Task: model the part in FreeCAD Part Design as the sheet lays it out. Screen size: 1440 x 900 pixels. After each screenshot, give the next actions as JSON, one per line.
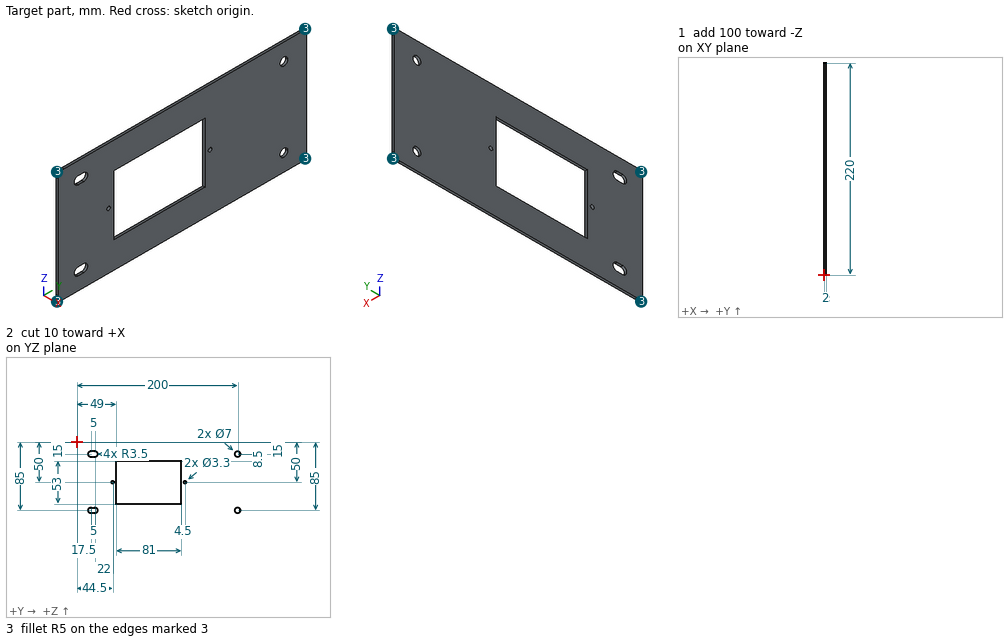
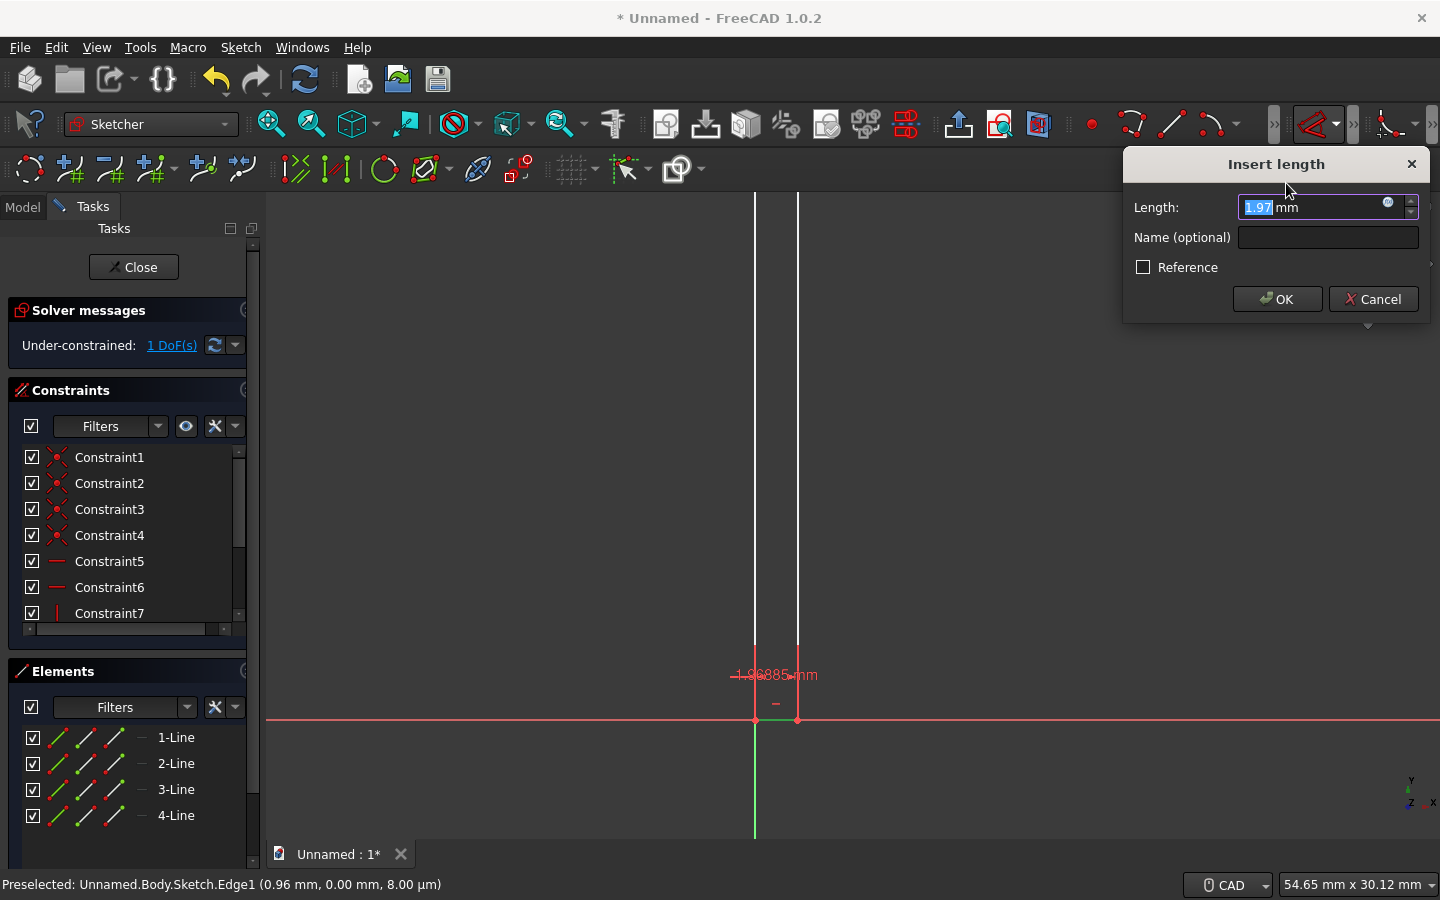
{"action": "type", "text": "2"}
{"action": "key", "text": "Return"}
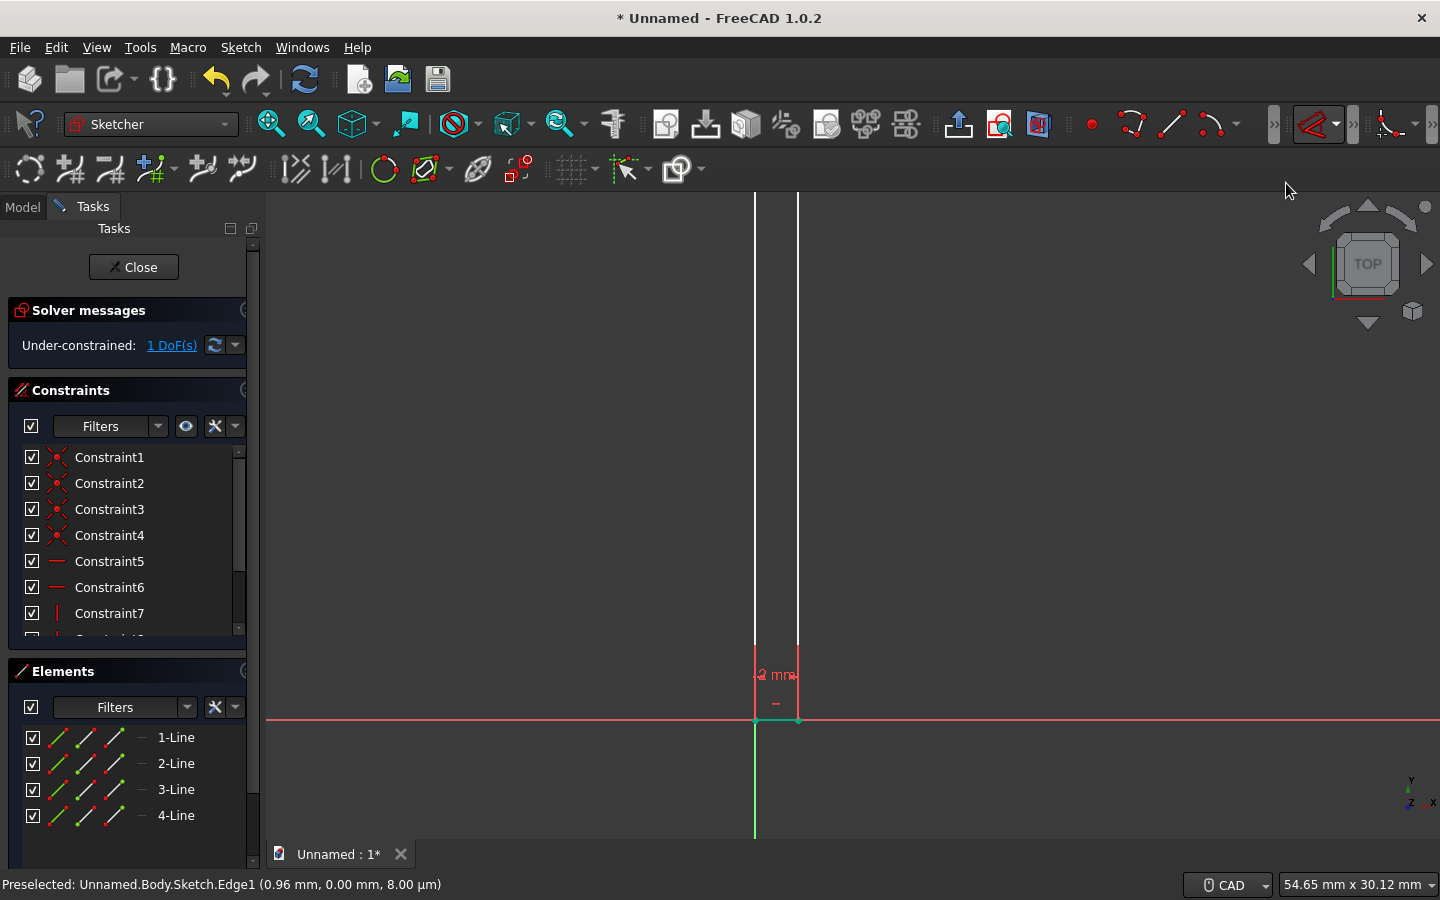
{"action": "scroll", "coordinate": [785, 731], "scroll_direction": "down", "scroll_amount": 12}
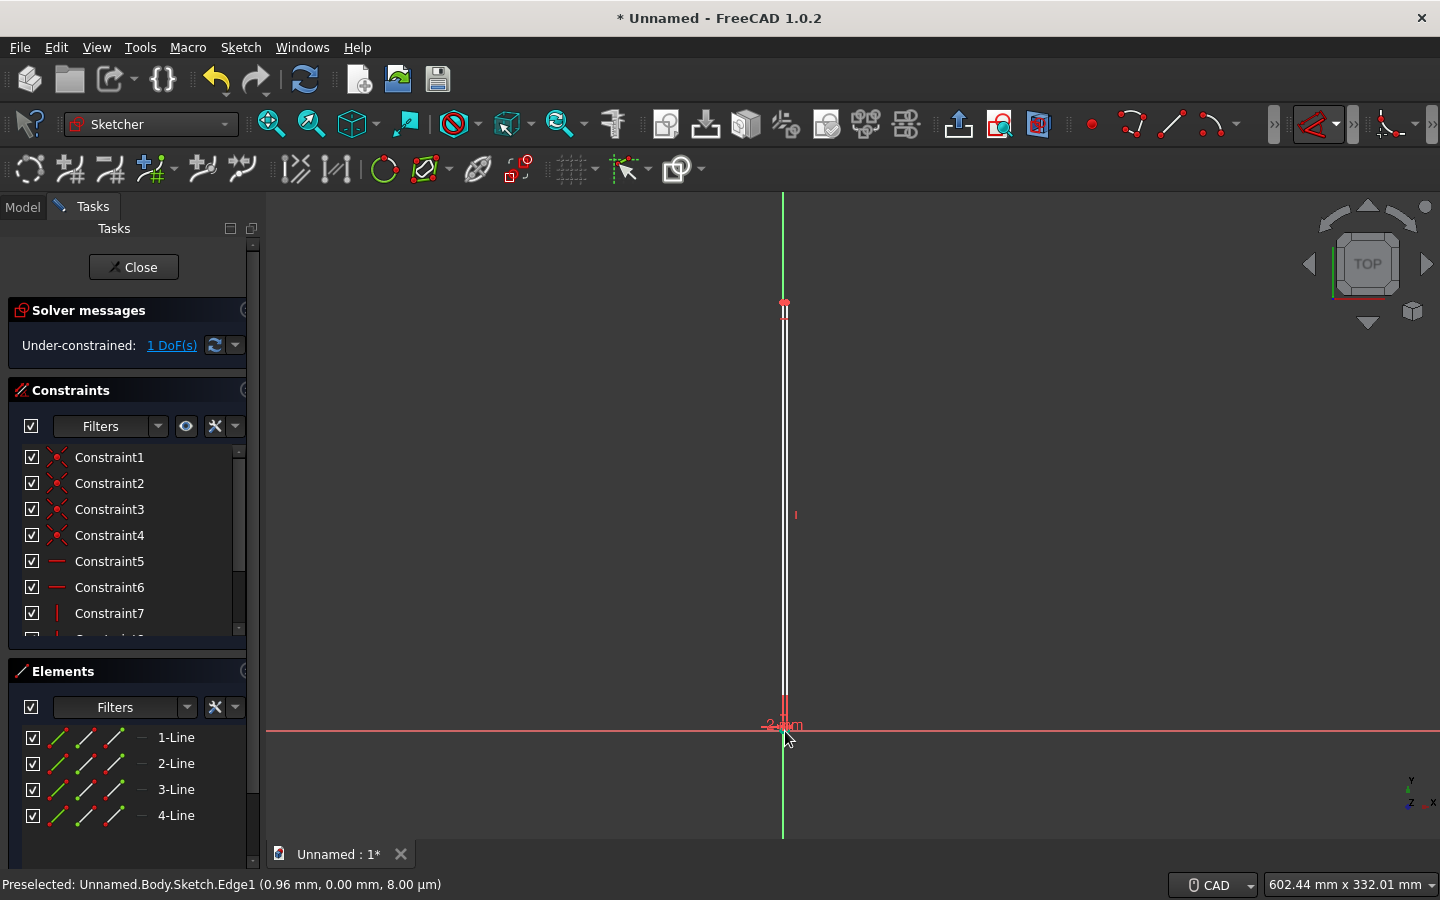
{"action": "scroll", "coordinate": [787, 602], "scroll_direction": "up", "scroll_amount": 7}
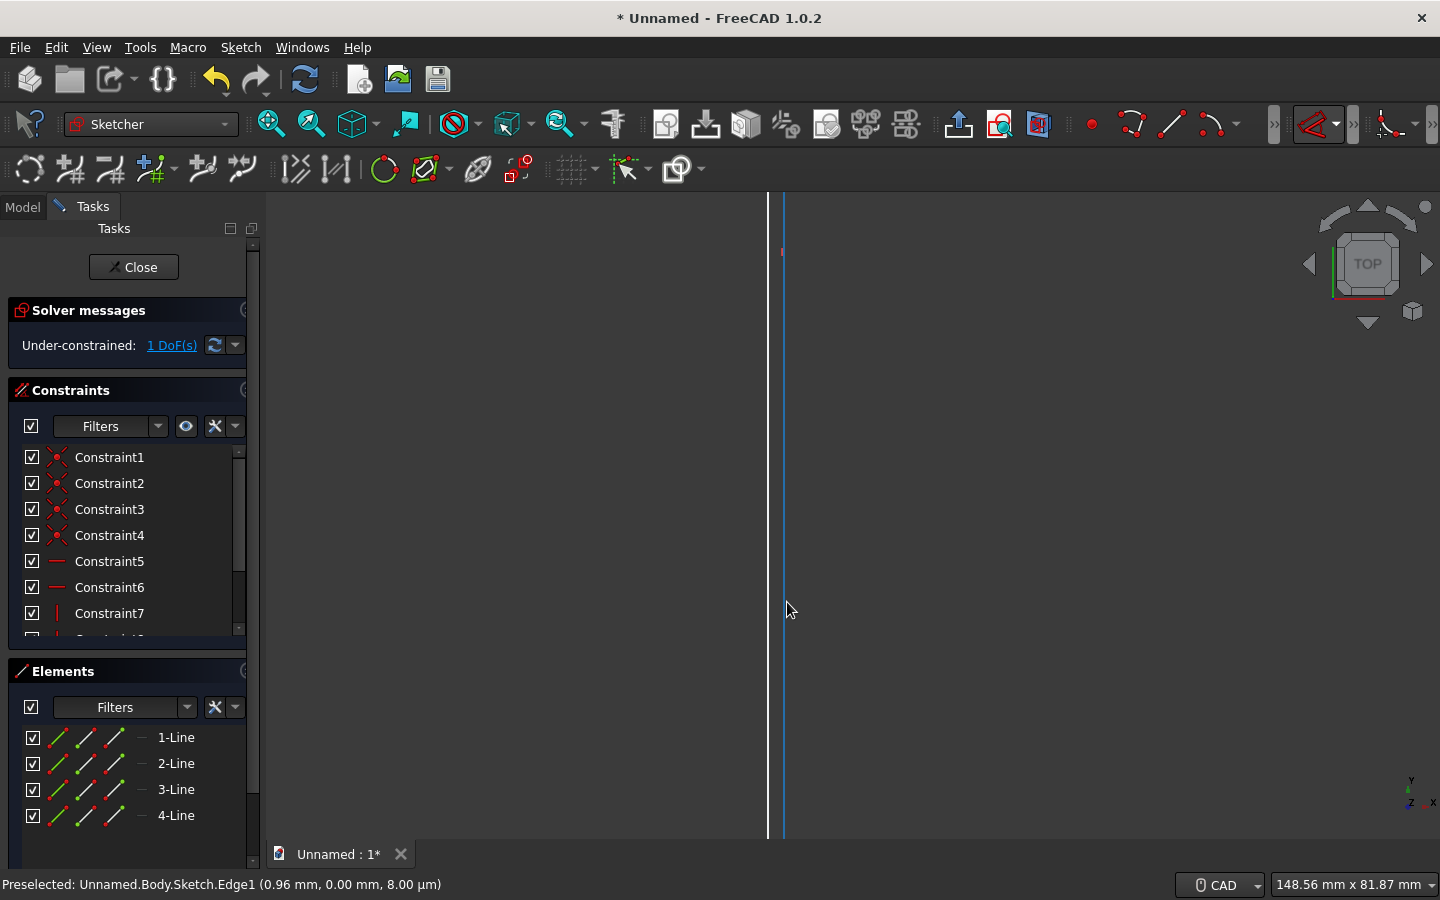
{"action": "left_click", "coordinate": [784, 601]}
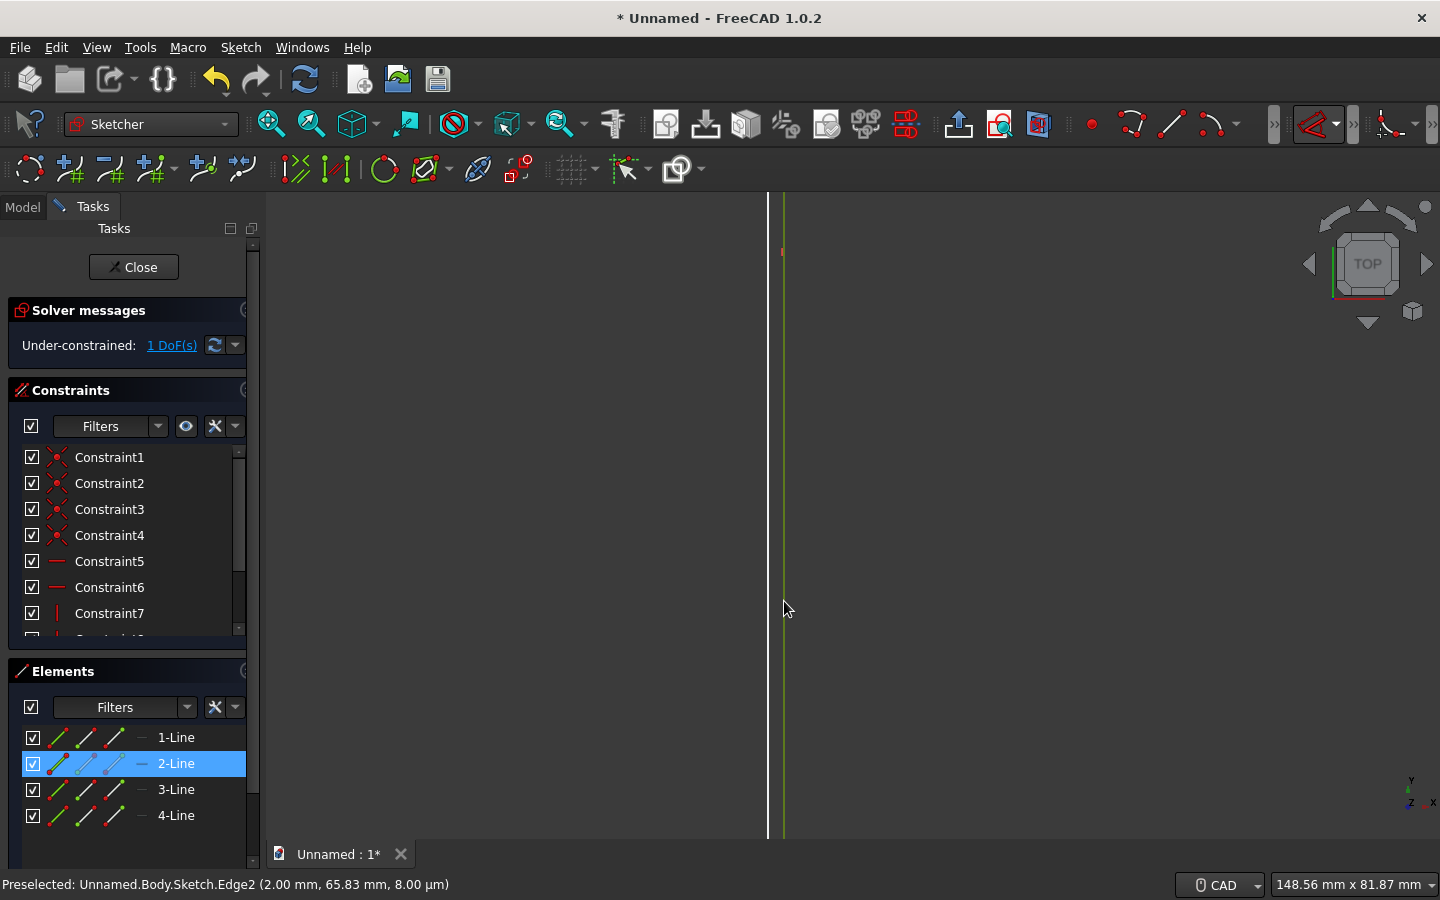
{"action": "left_click", "coordinate": [1338, 124]}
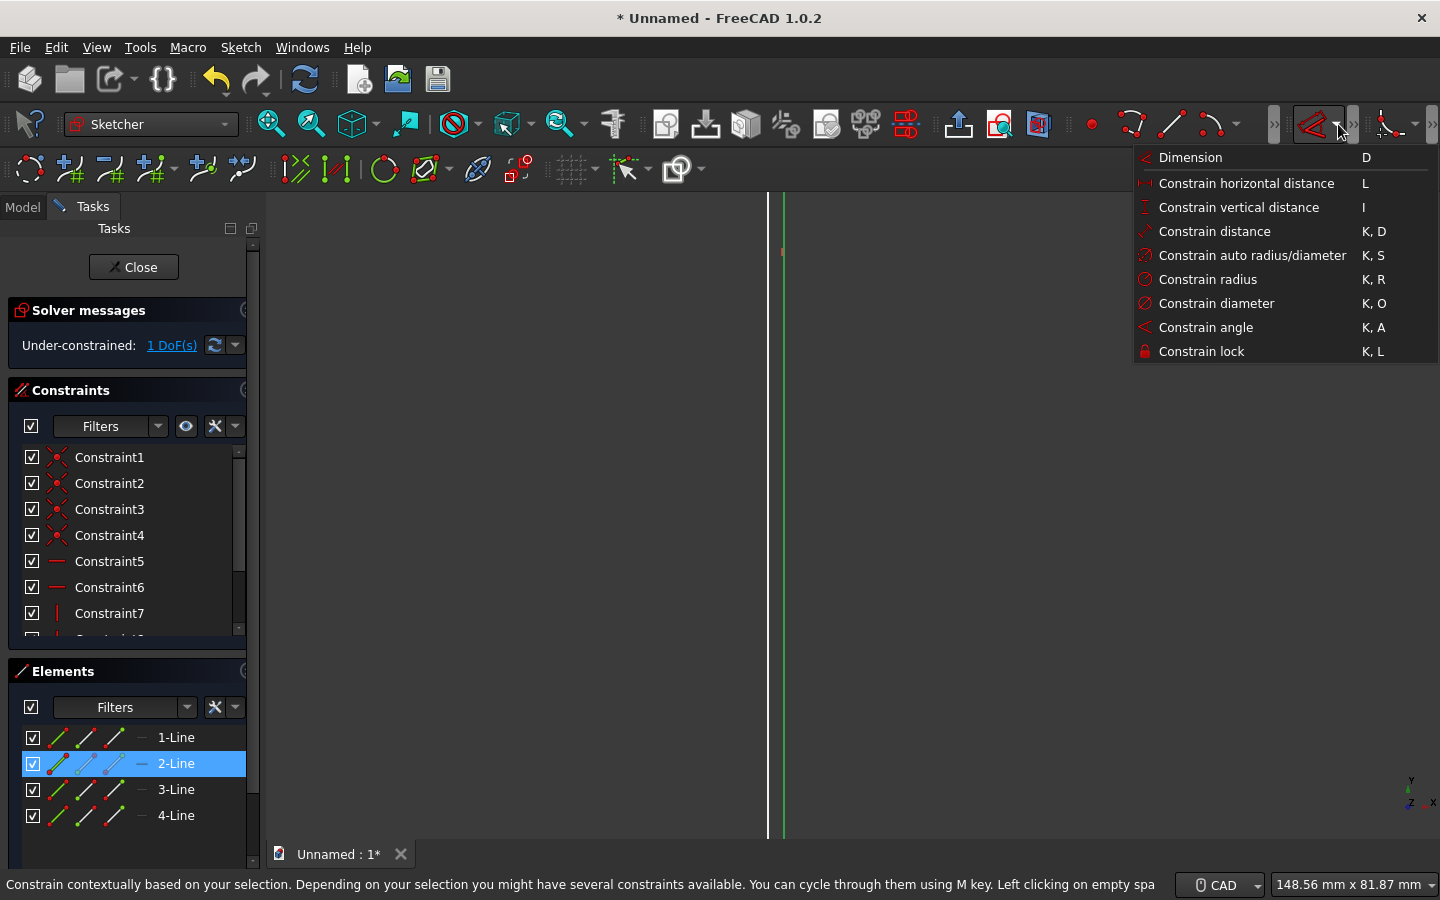
{"action": "left_click", "coordinate": [1286, 207]}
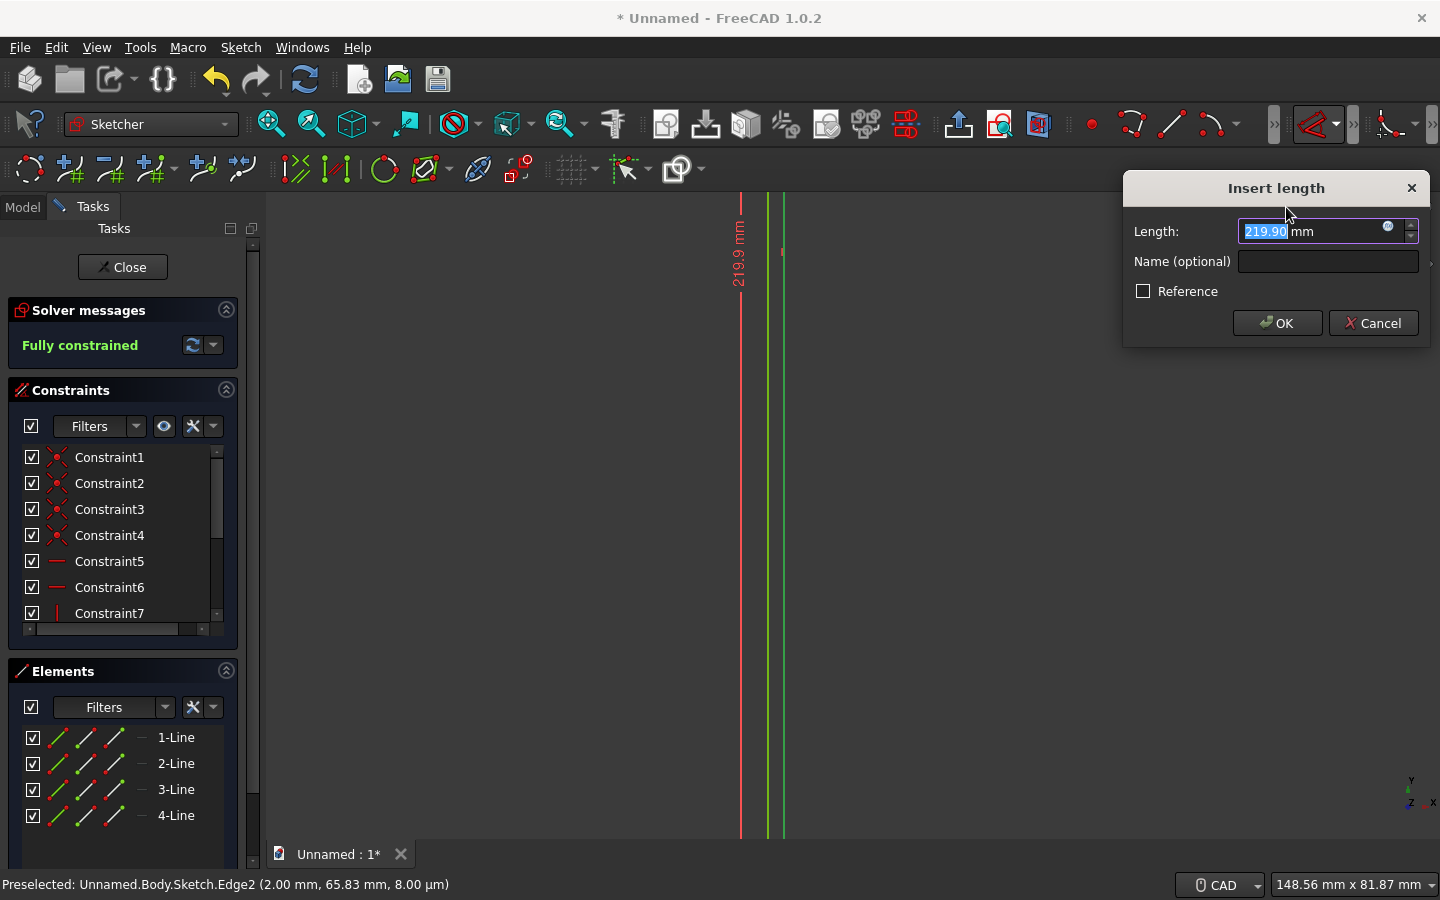
{"action": "type", "text": "220"}
{"action": "key", "text": "Return"}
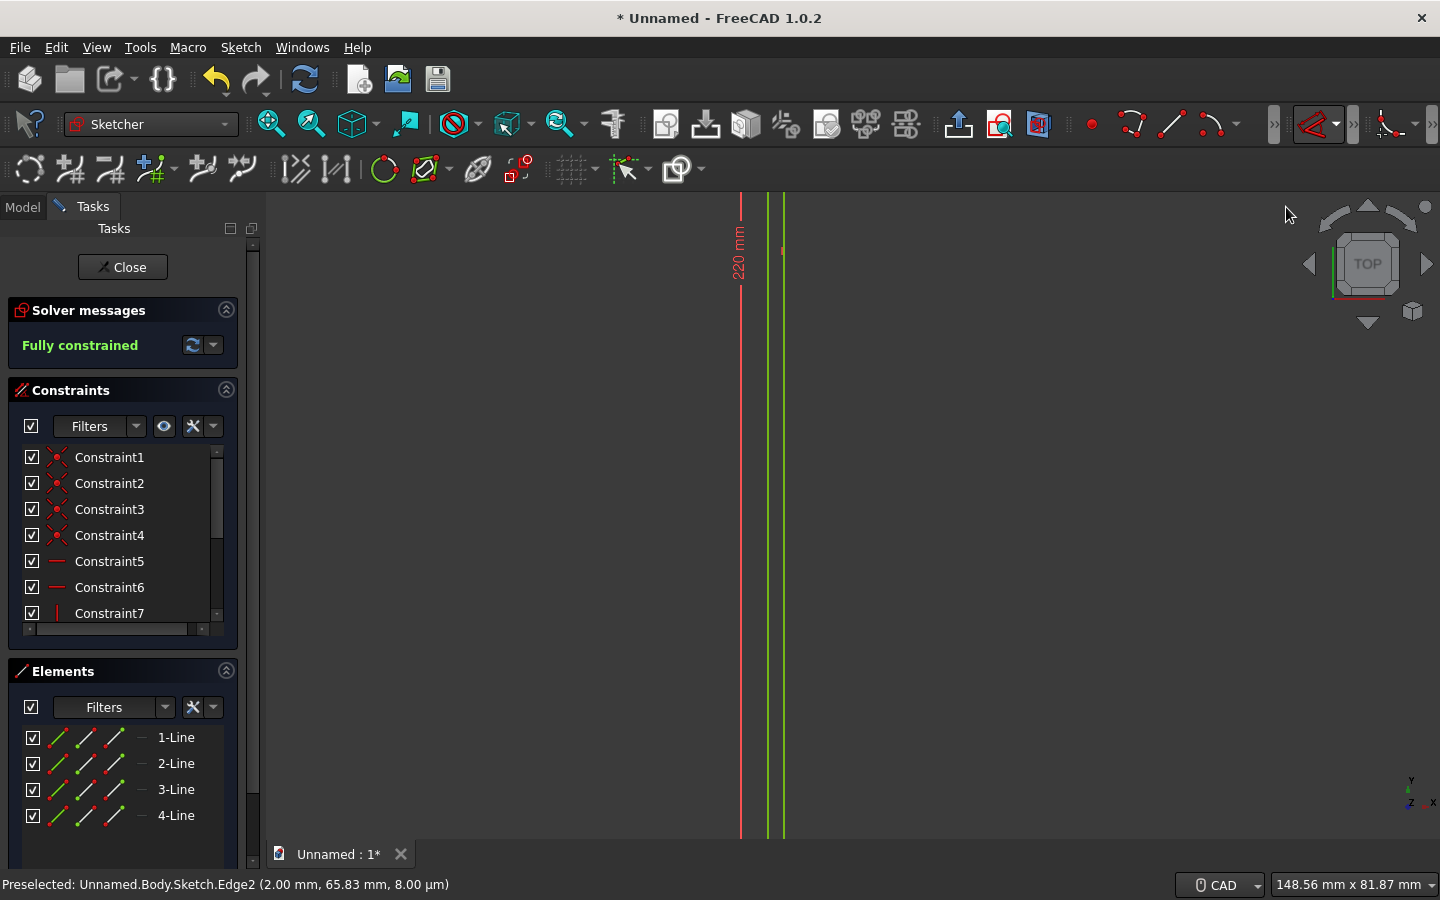
{"action": "left_click", "coordinate": [123, 267]}